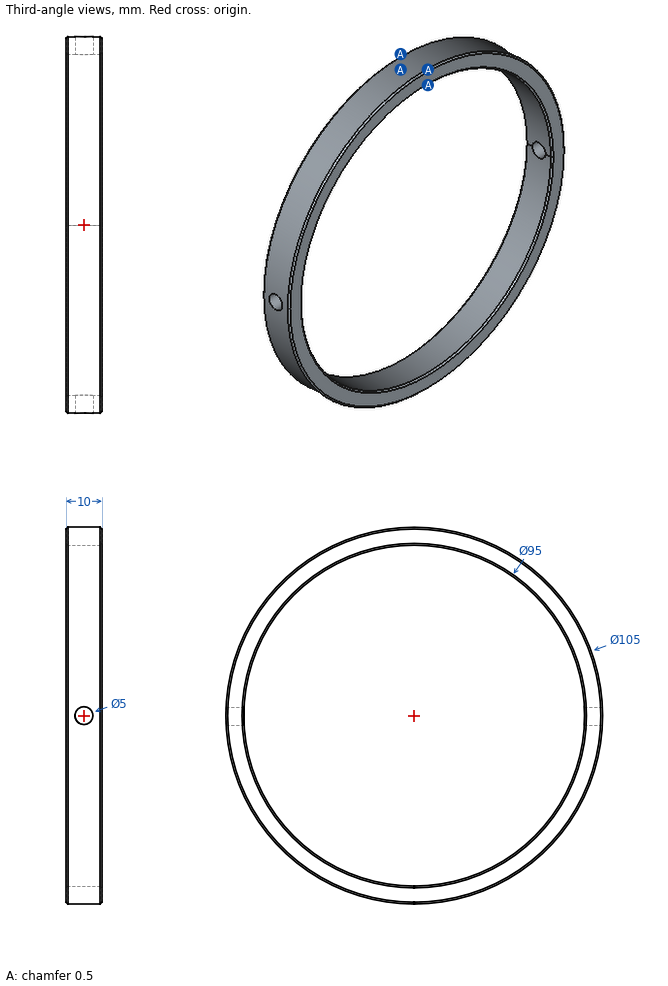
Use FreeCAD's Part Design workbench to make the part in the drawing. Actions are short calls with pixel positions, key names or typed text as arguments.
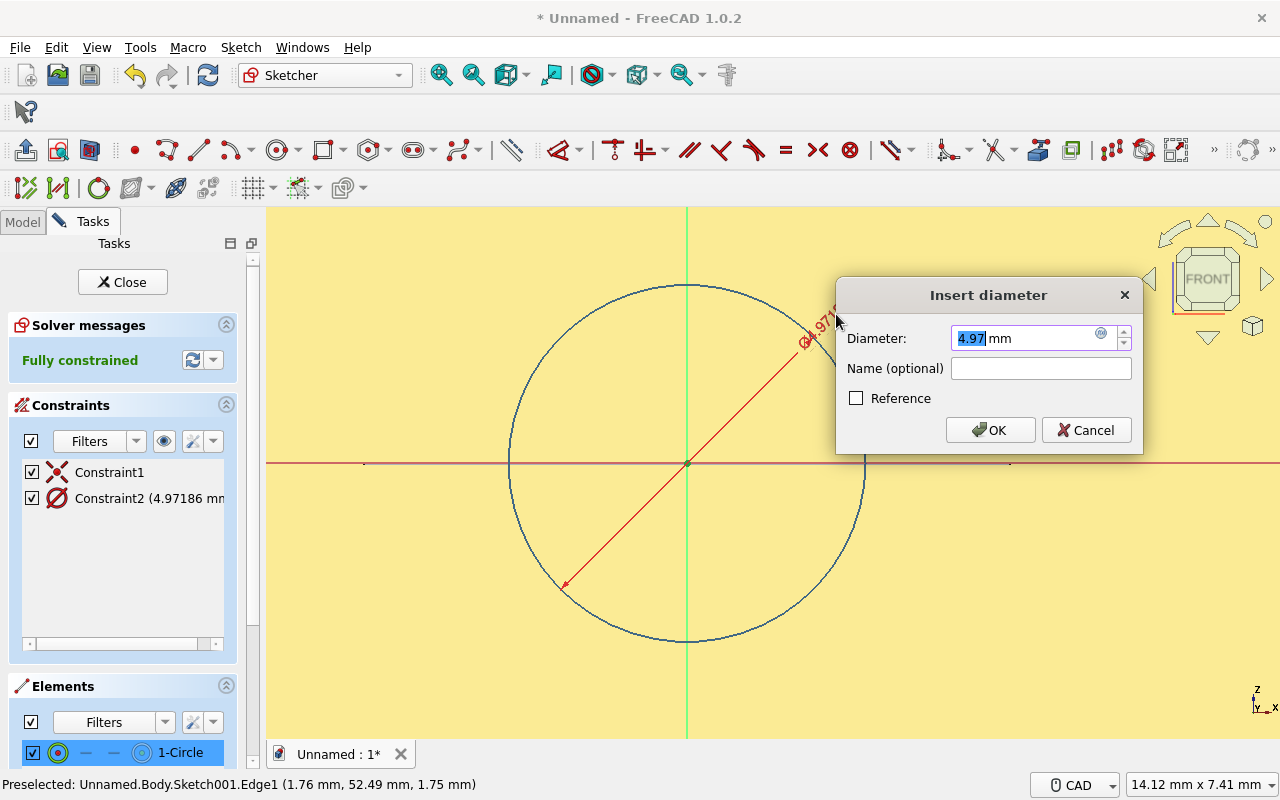
text(5)
key(Return)
key(Escape)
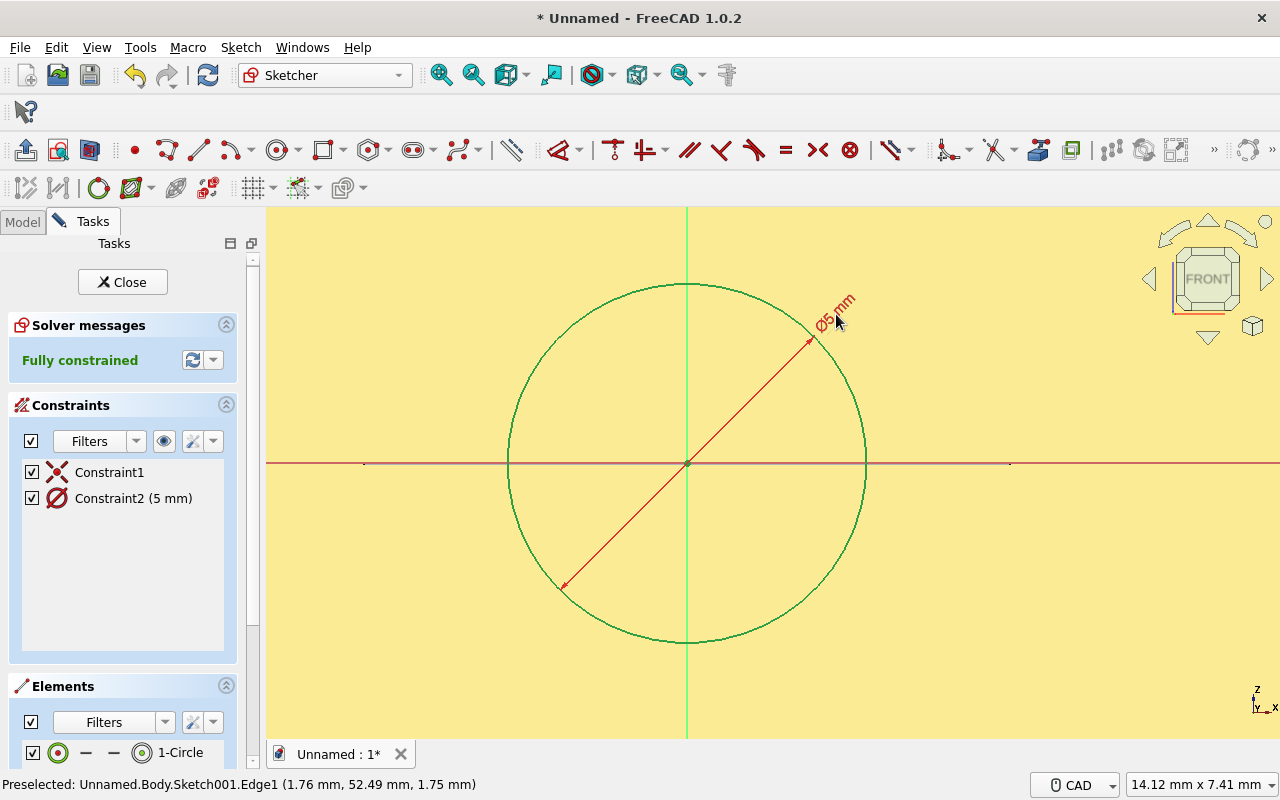
click(123, 282)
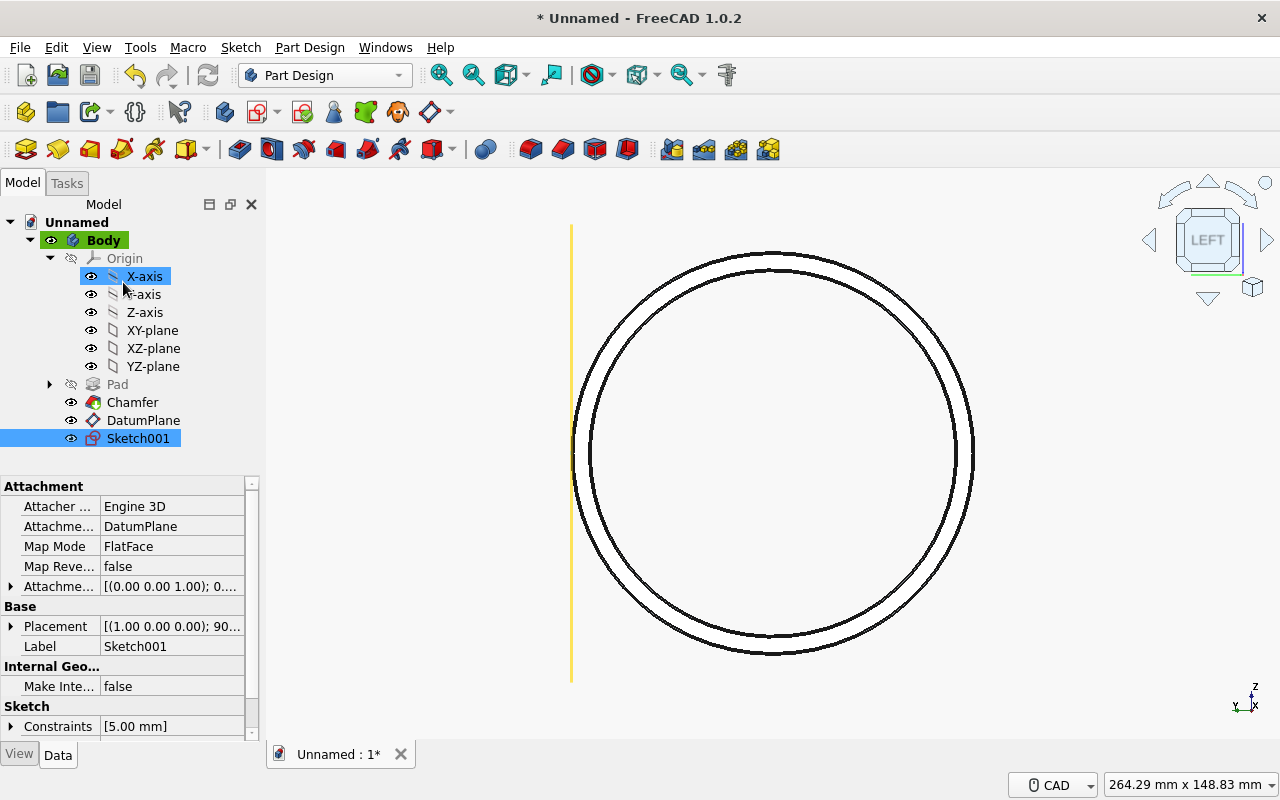
click(240, 150)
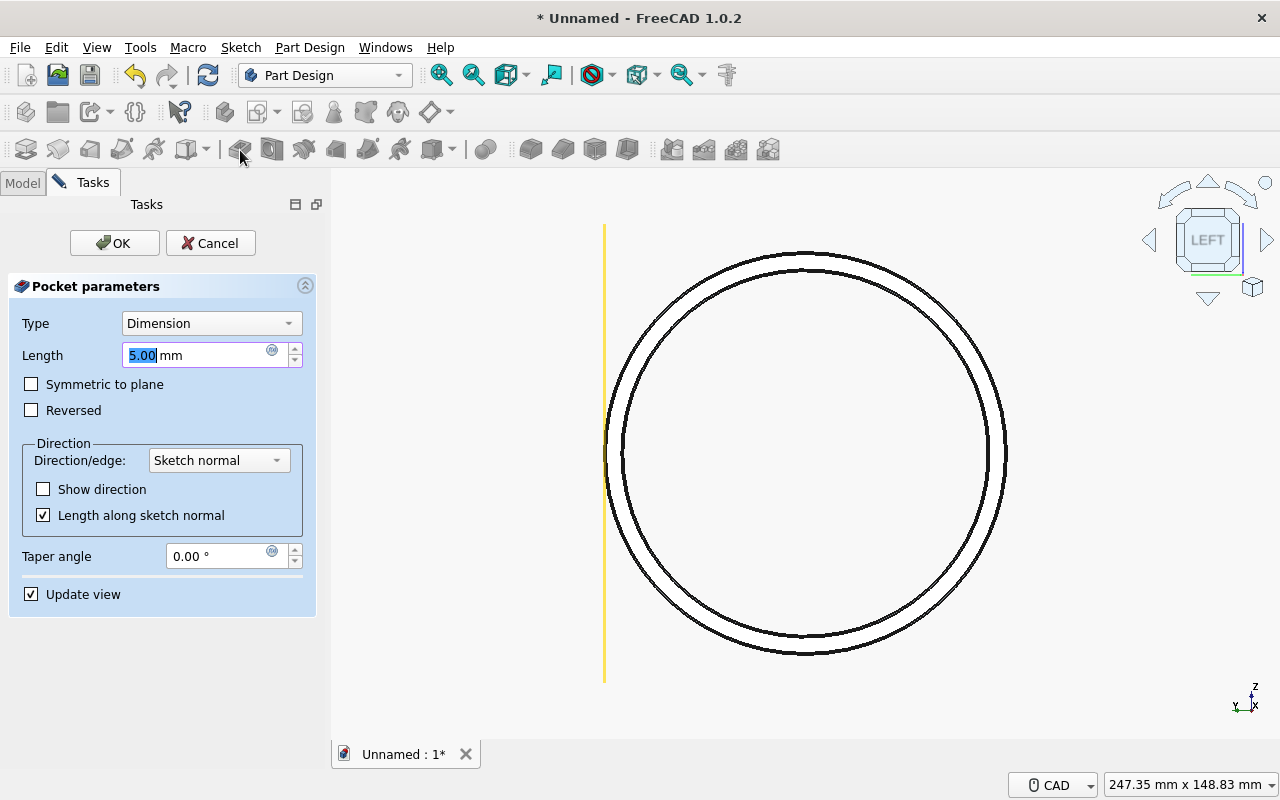
click(212, 324)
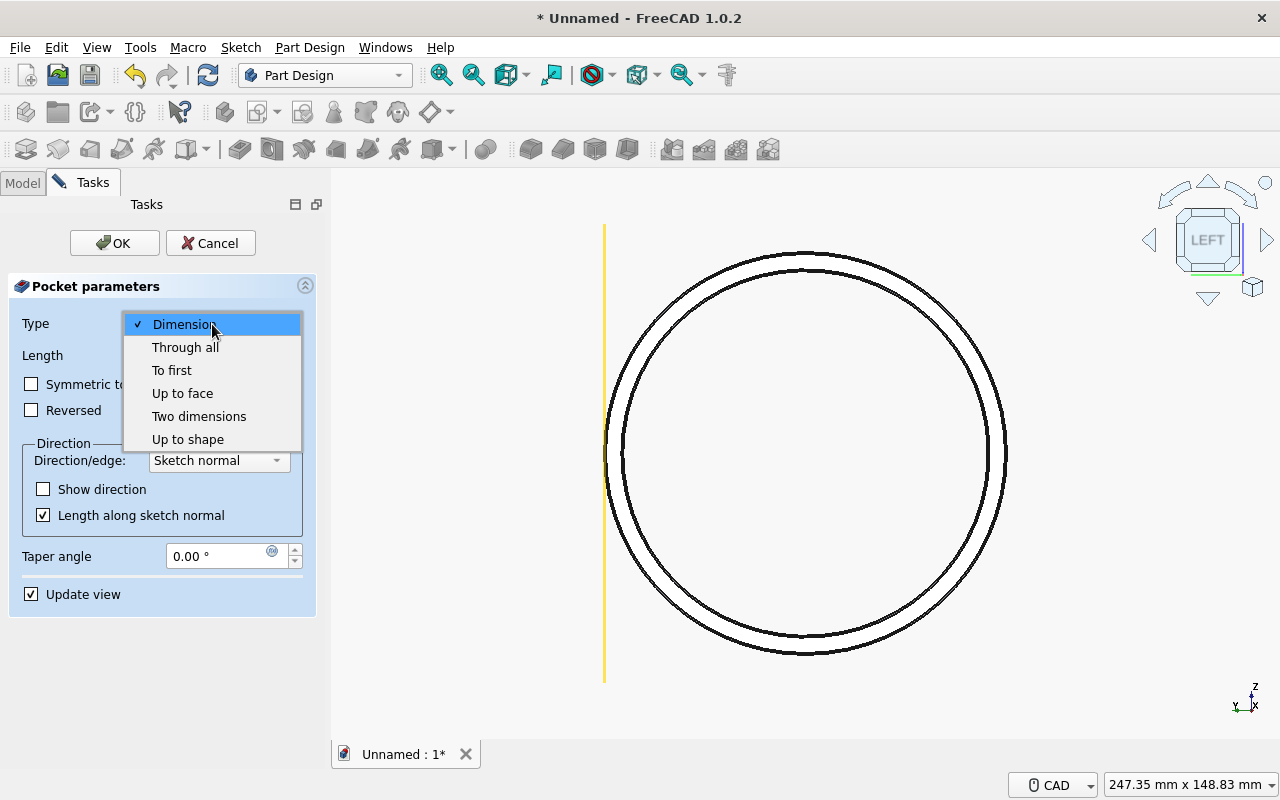
click(212, 348)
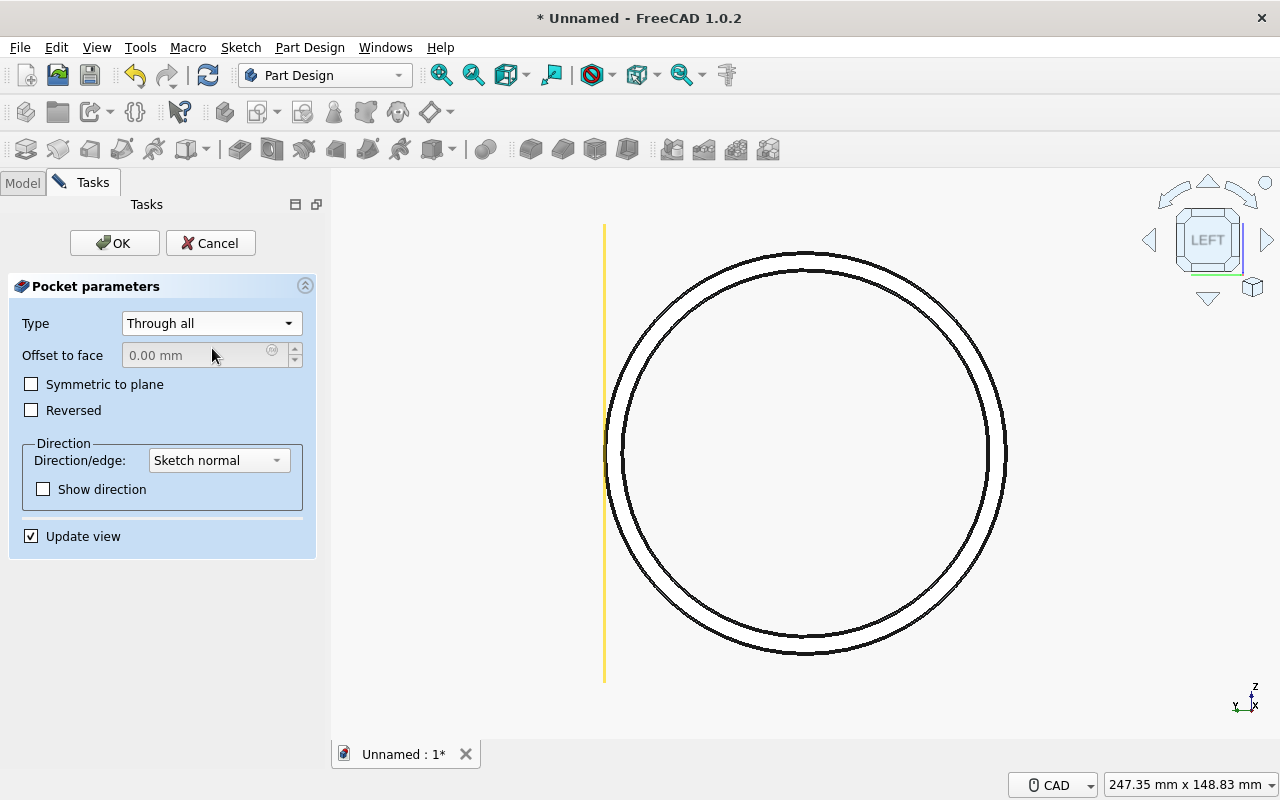
click(30, 410)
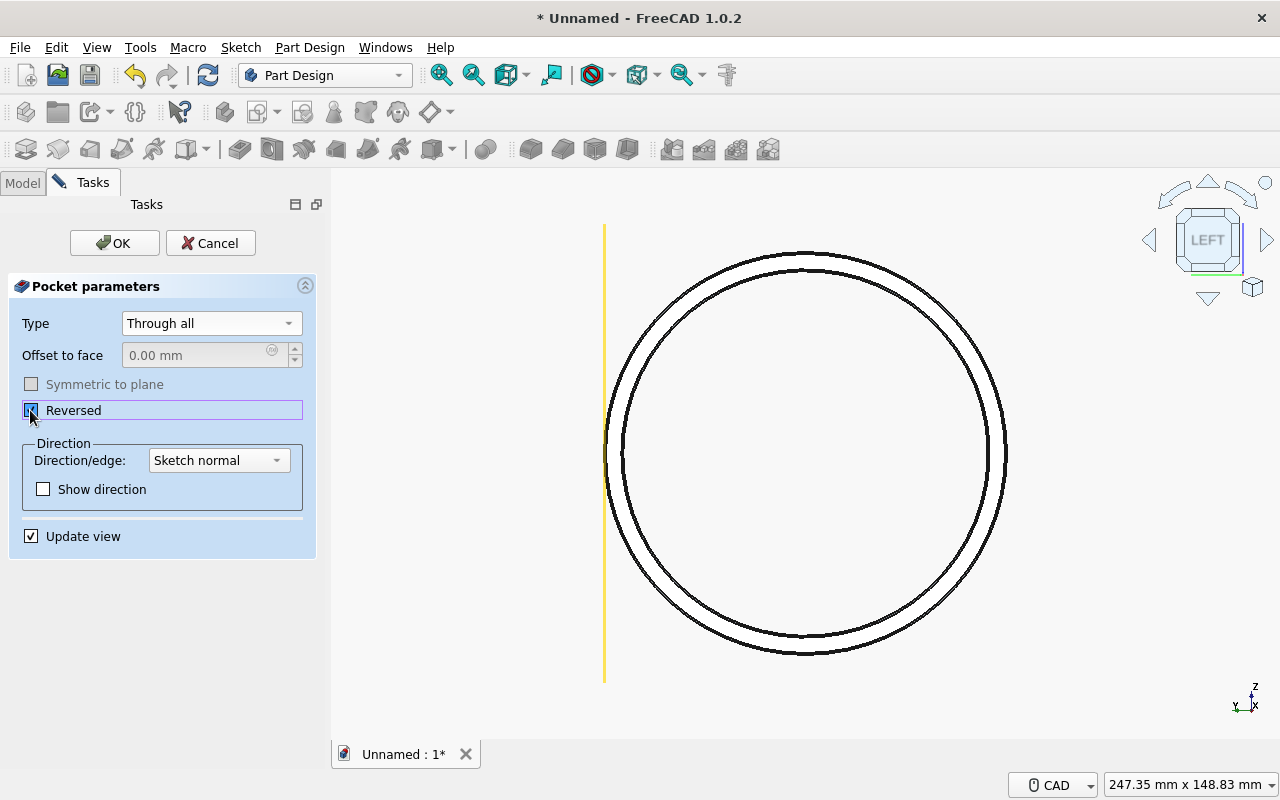
click(115, 243)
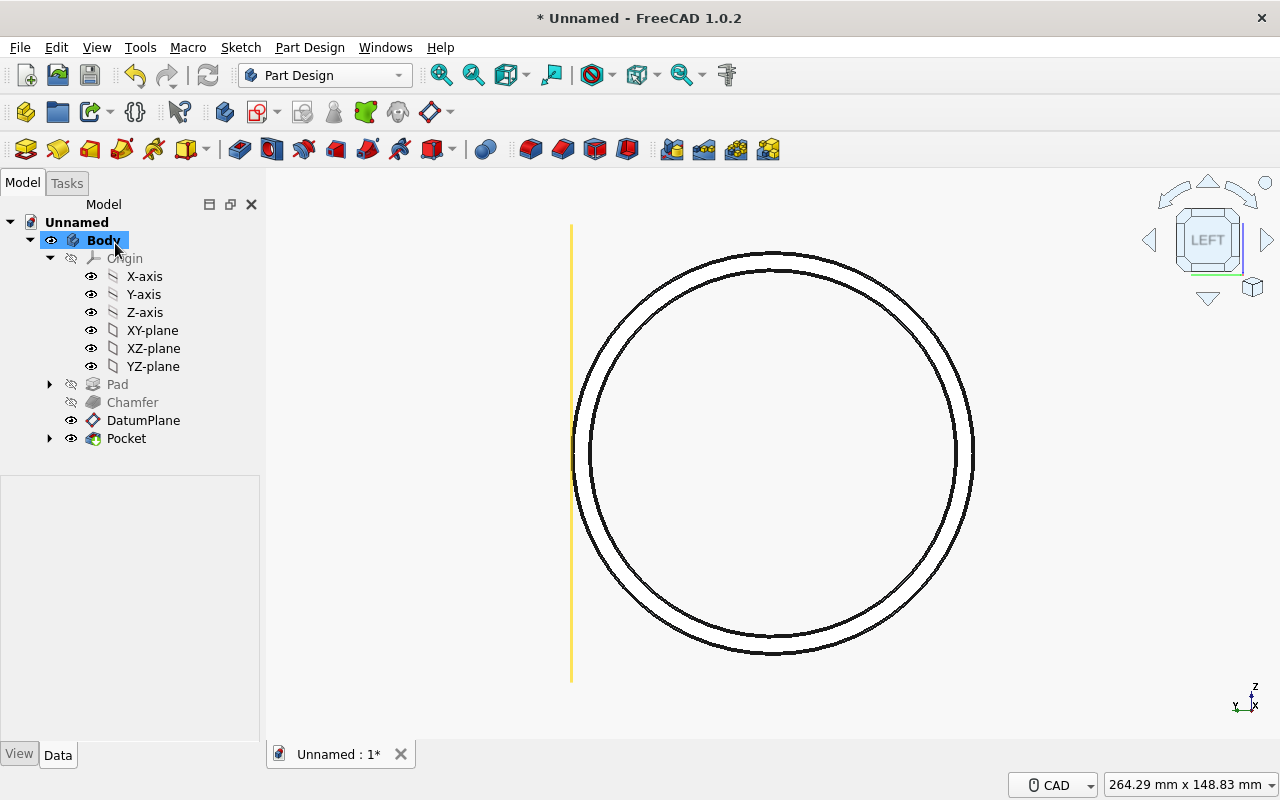
click(116, 420)
key(space)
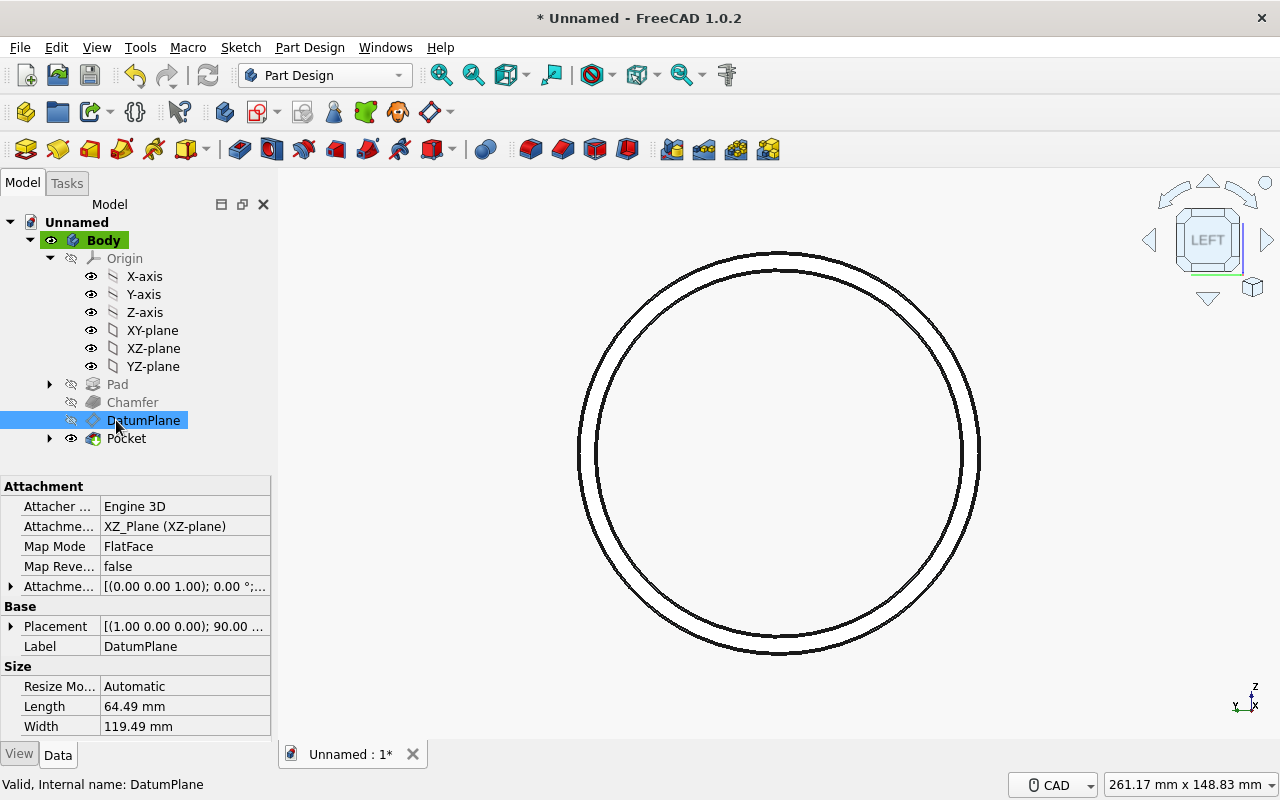
key(0)